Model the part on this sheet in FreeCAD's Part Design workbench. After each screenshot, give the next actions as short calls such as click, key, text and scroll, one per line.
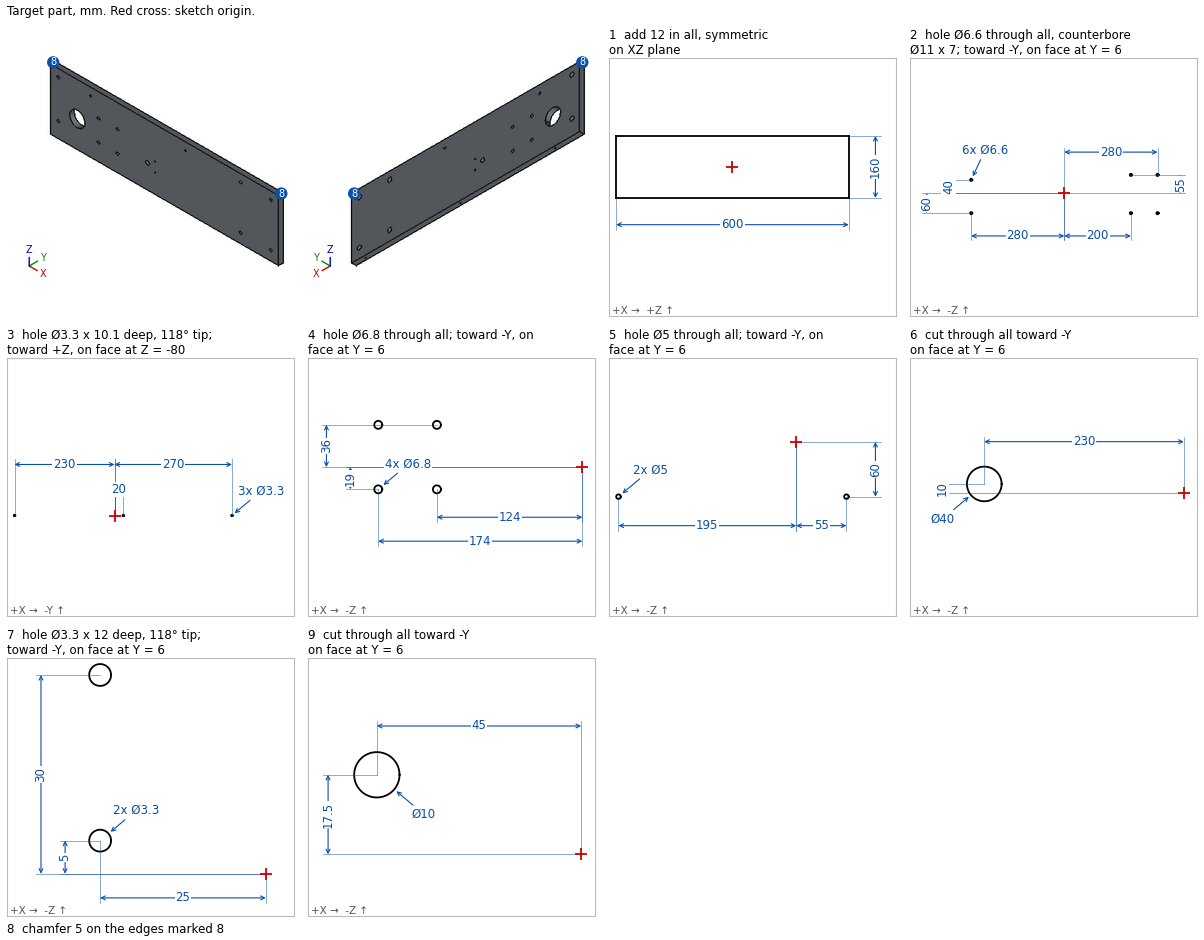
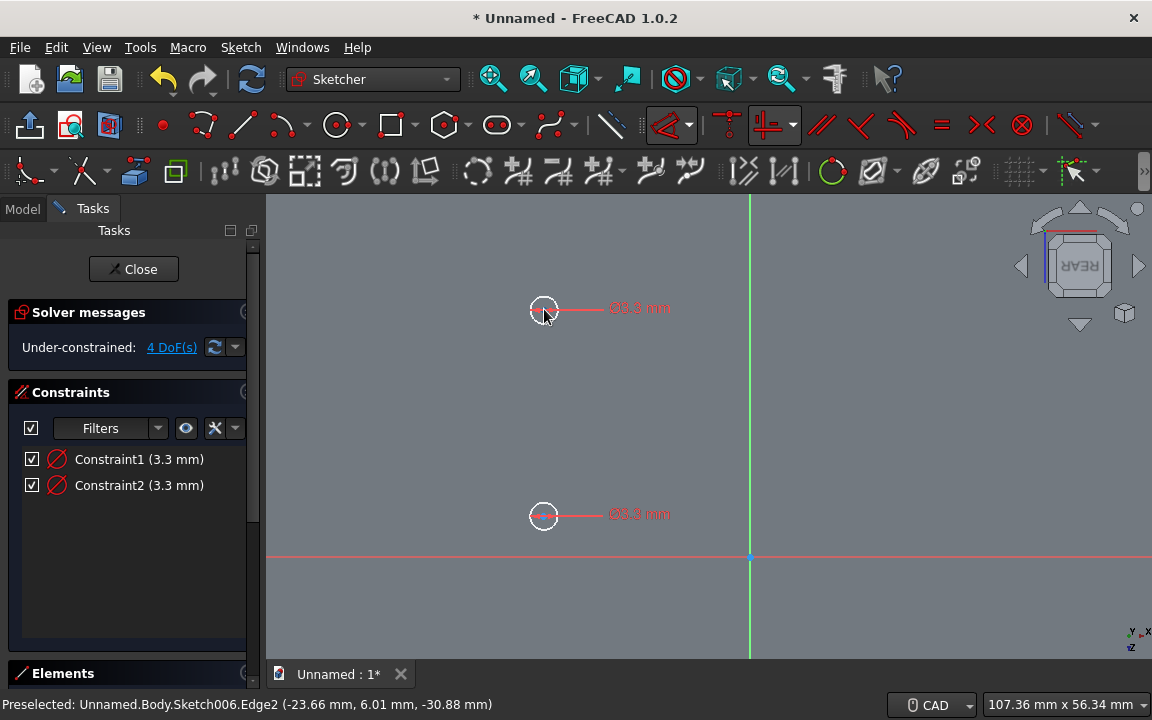
click(544, 516)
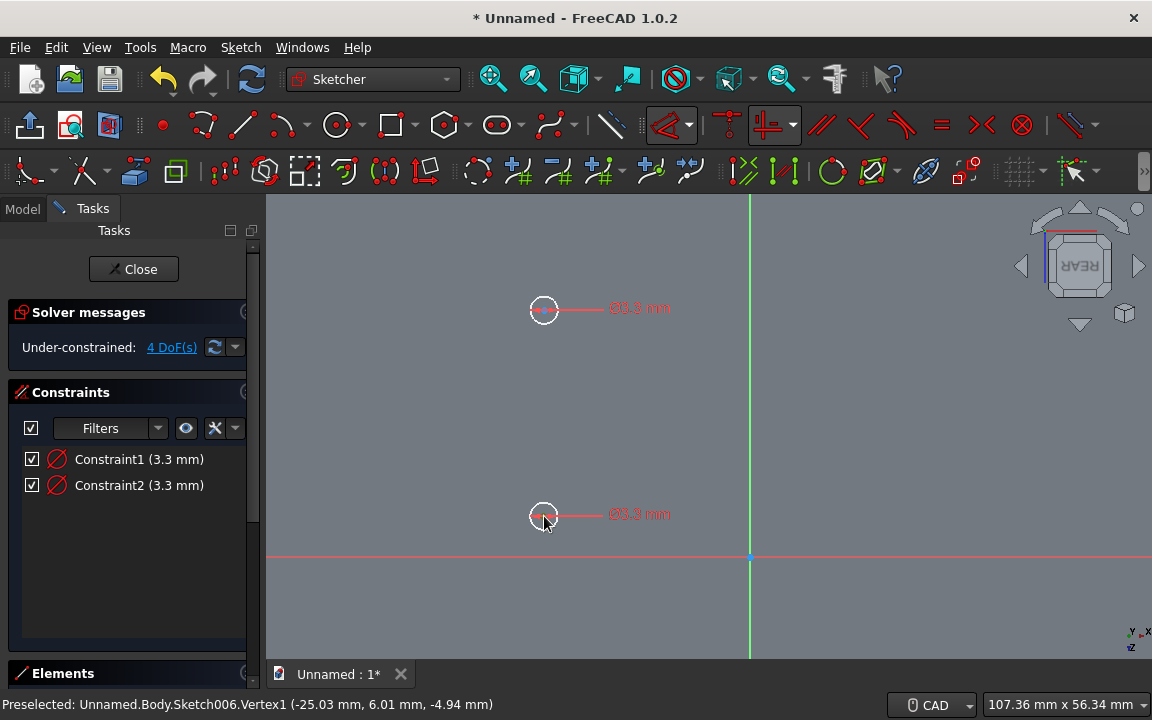
click(544, 310)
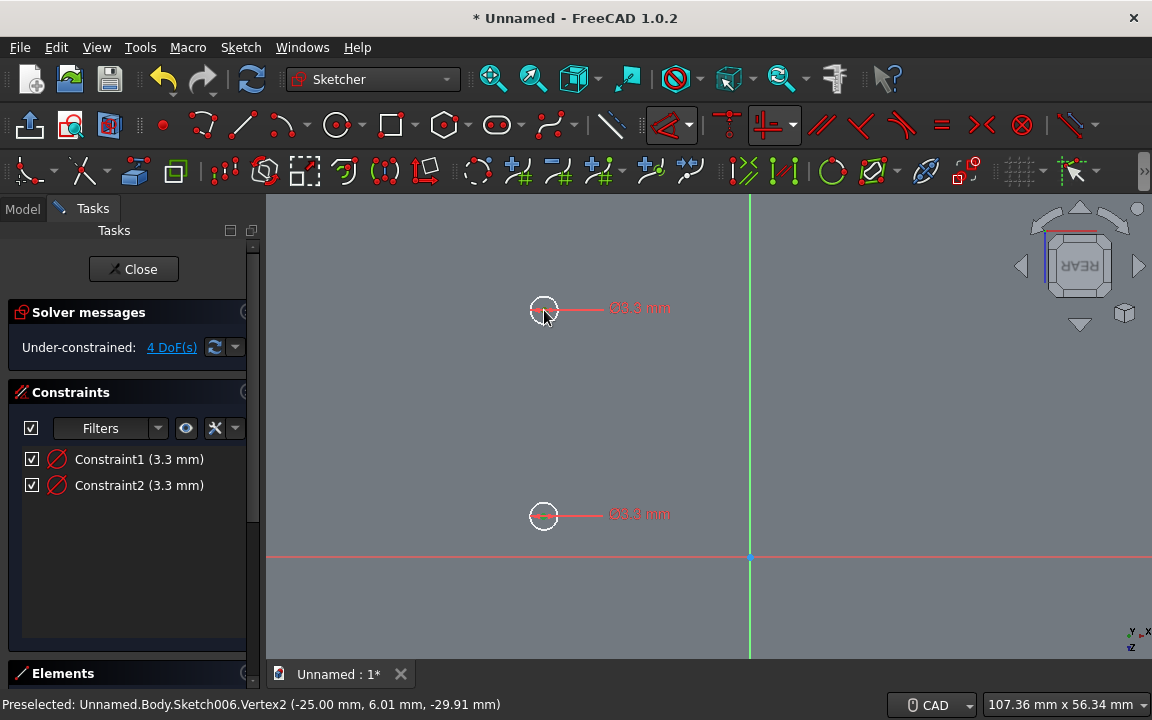
click(796, 126)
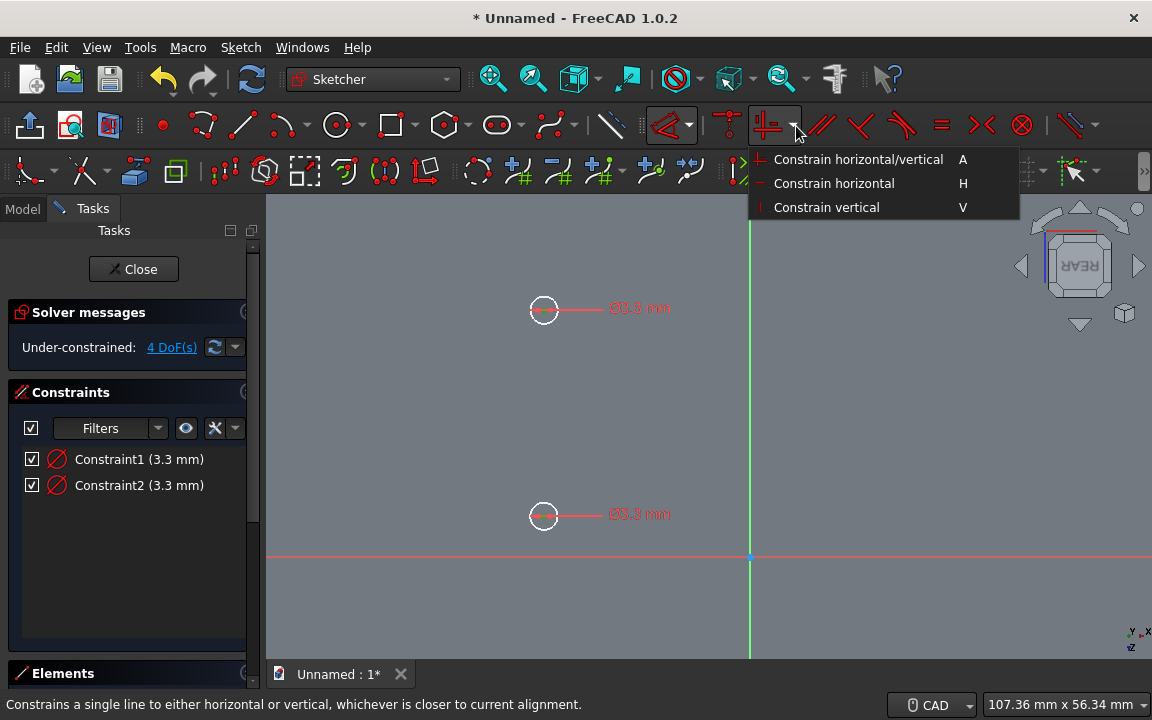
click(884, 207)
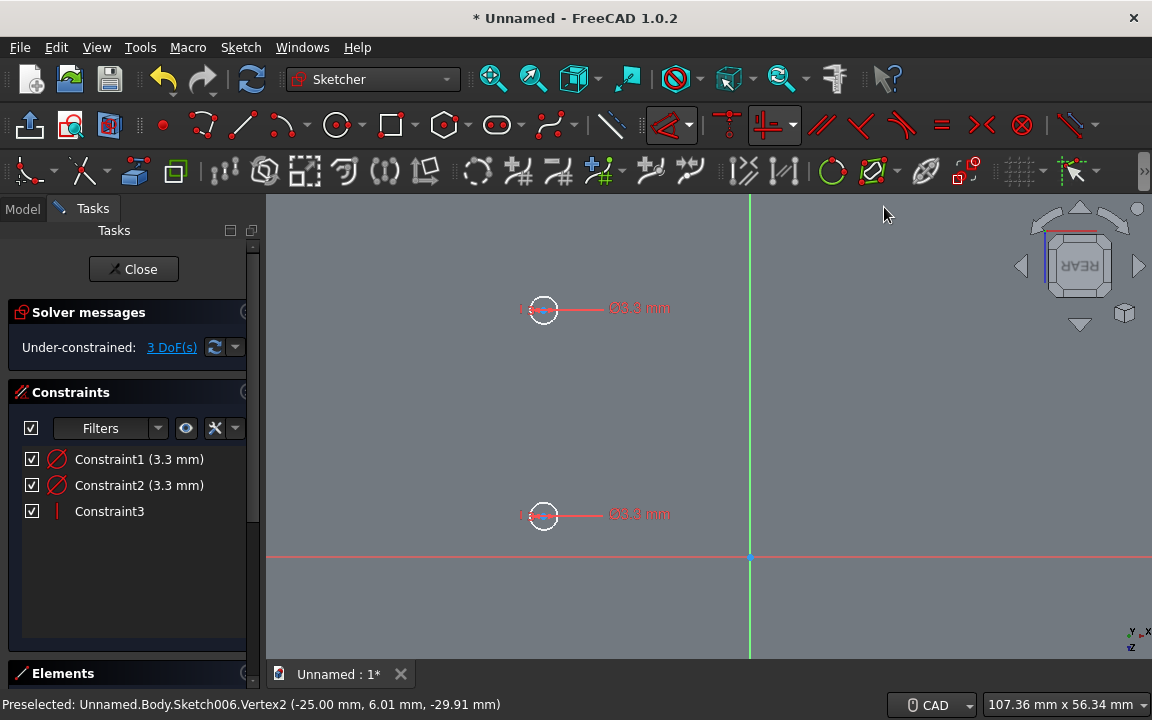
click(544, 516)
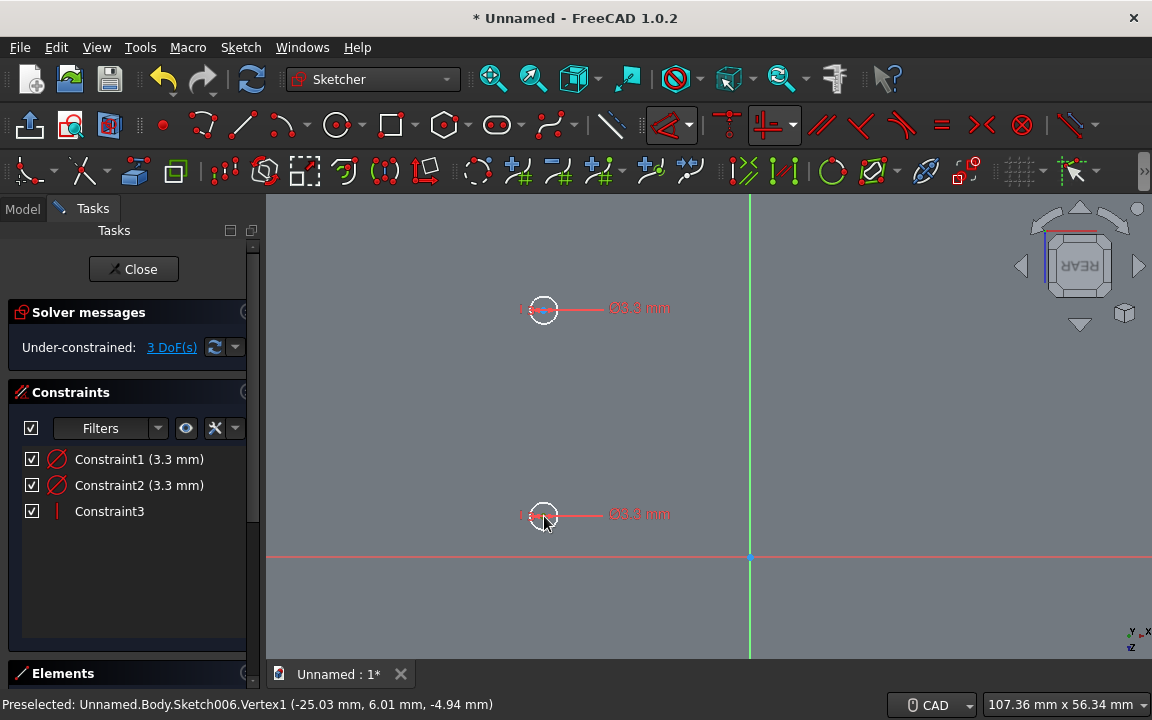
key(i)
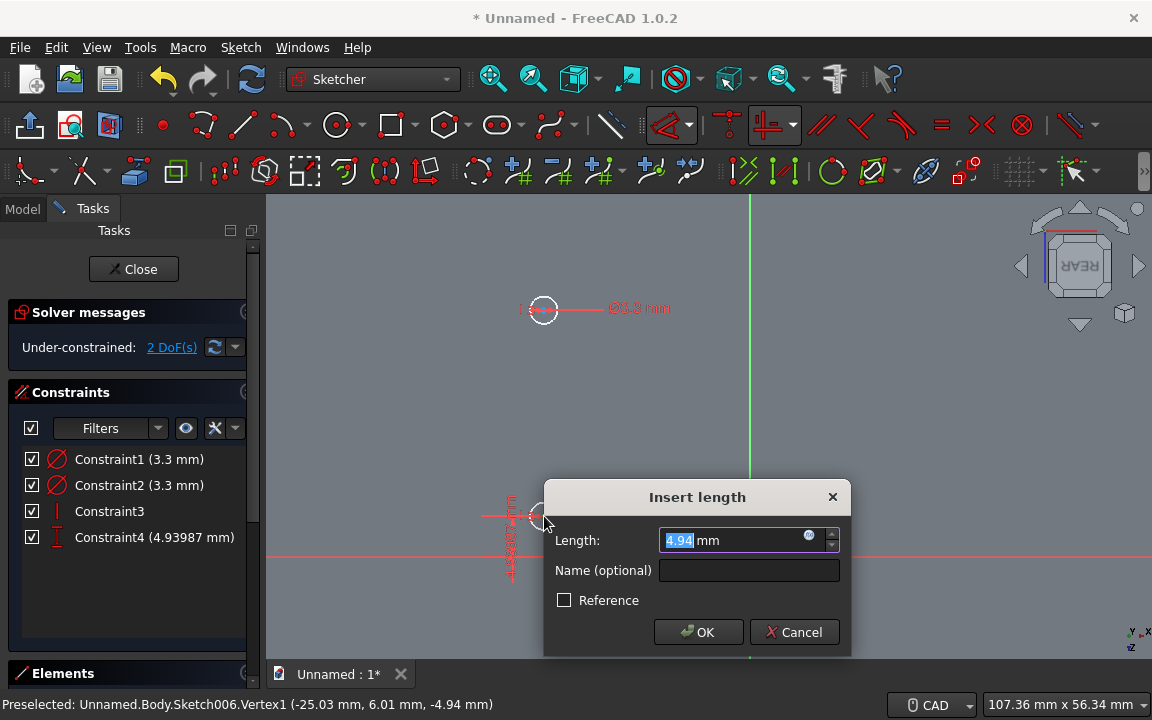
text(5)
key(Return)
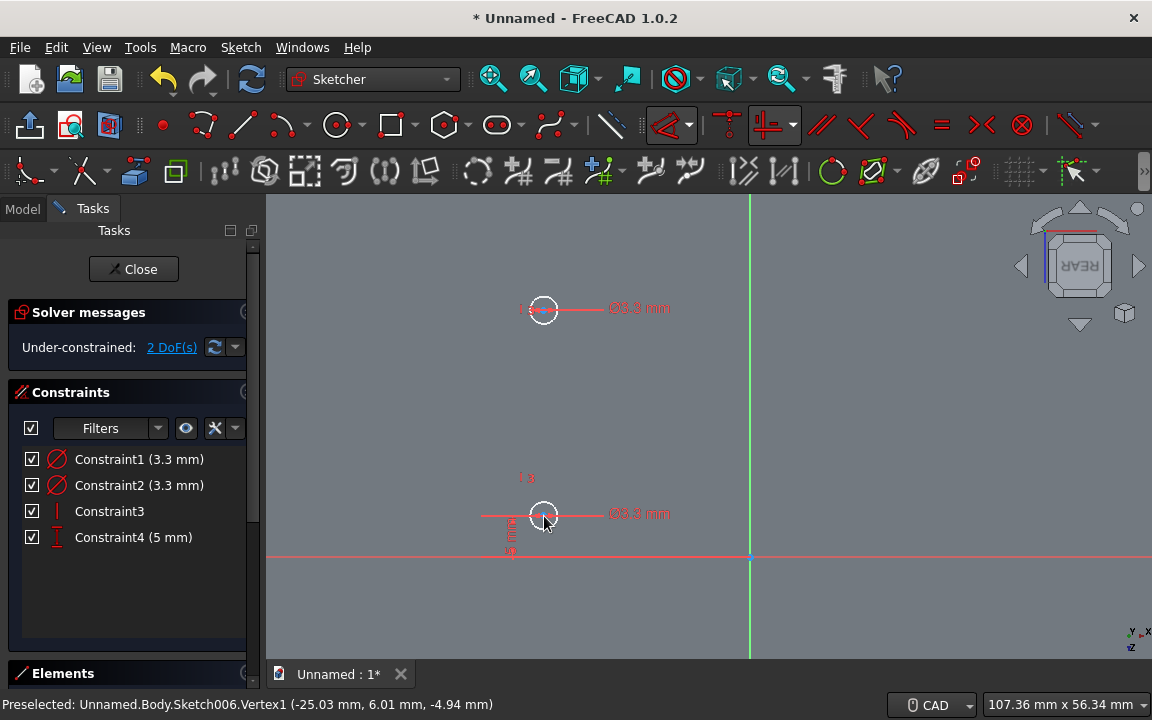
click(544, 516)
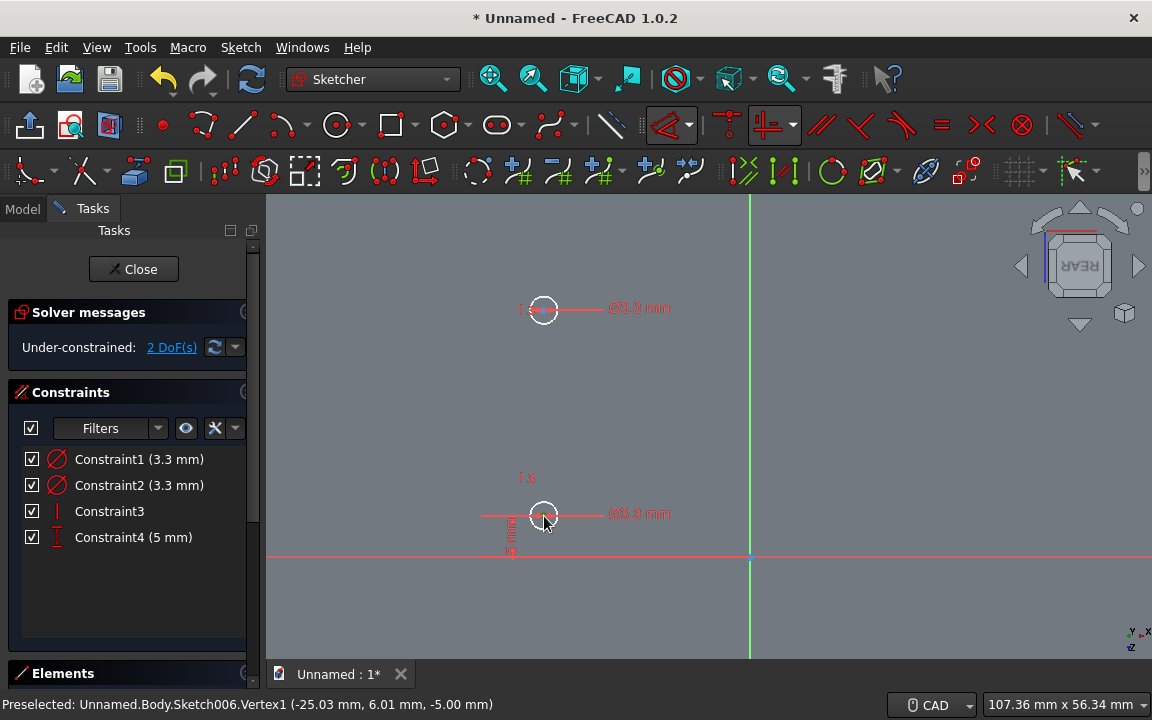
click(692, 126)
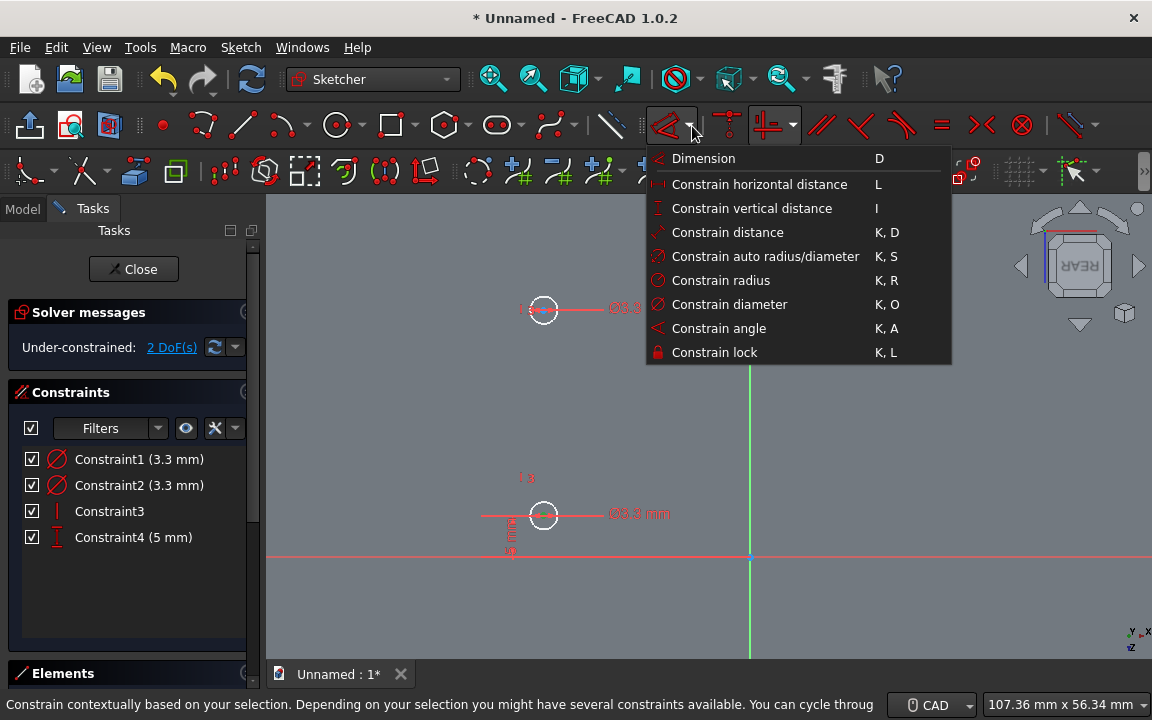
click(799, 184)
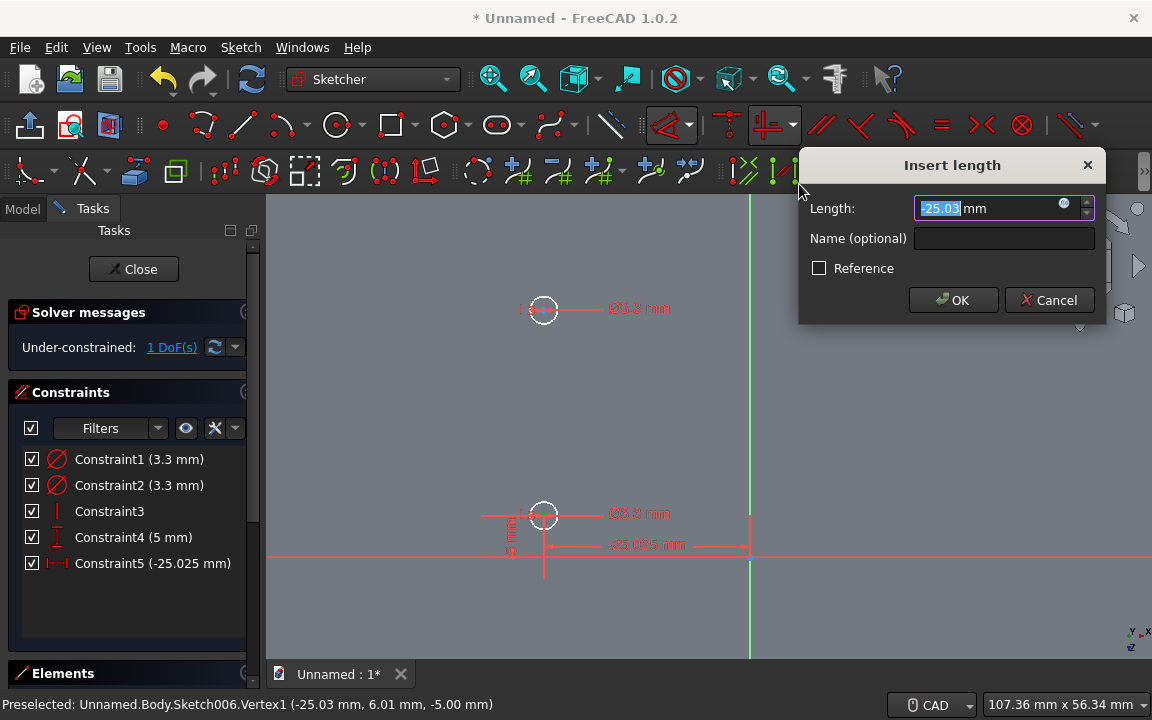
text(-25)
key(Return)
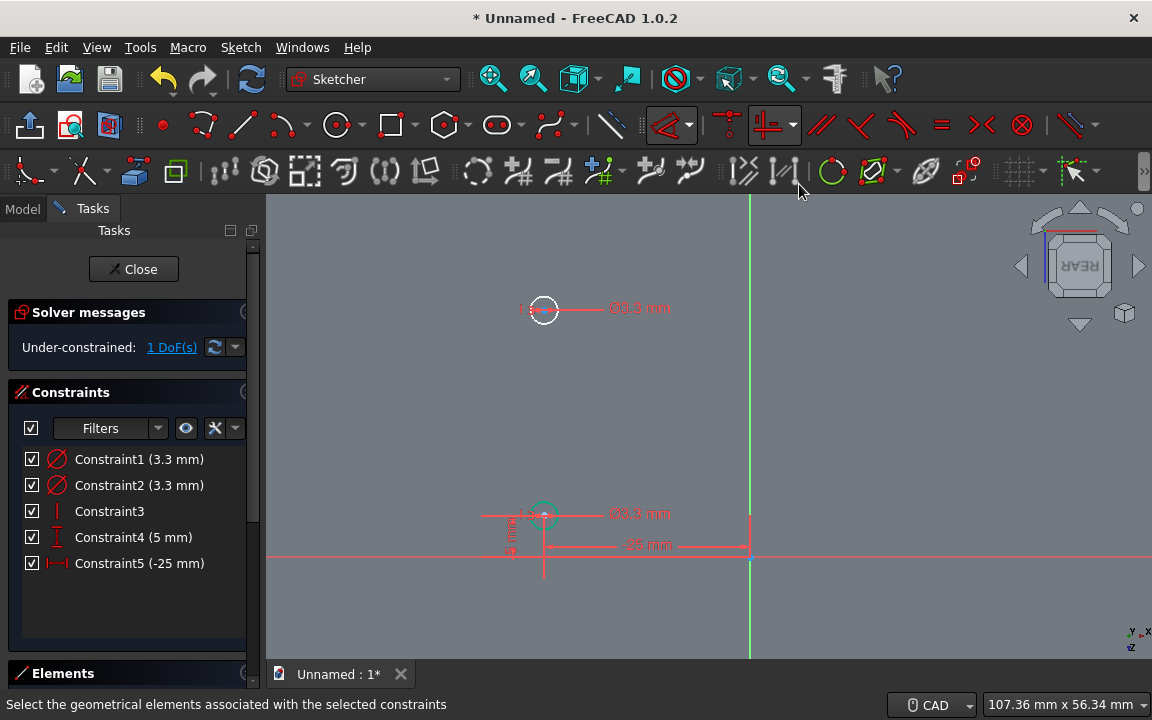
click(544, 310)